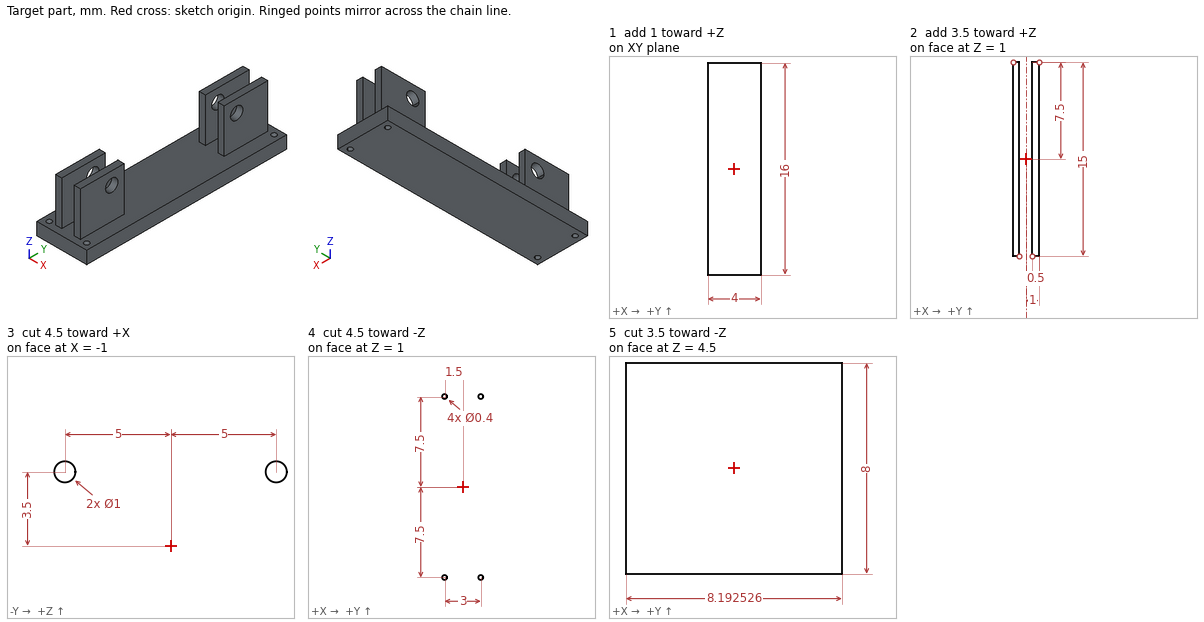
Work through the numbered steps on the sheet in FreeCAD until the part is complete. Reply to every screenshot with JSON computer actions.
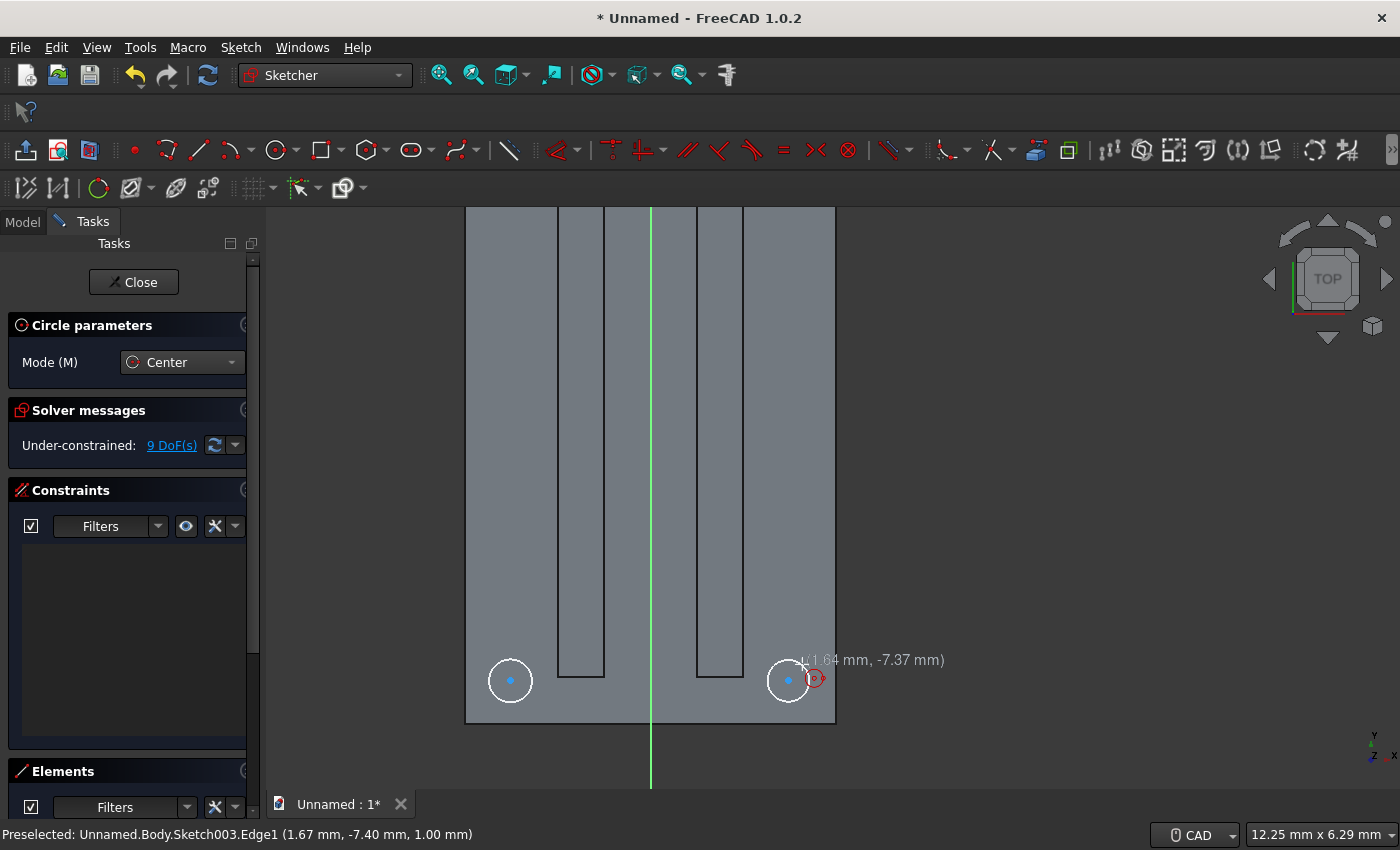
{"action": "scroll", "coordinate": [802, 666], "scroll_direction": "down", "scroll_amount": 7}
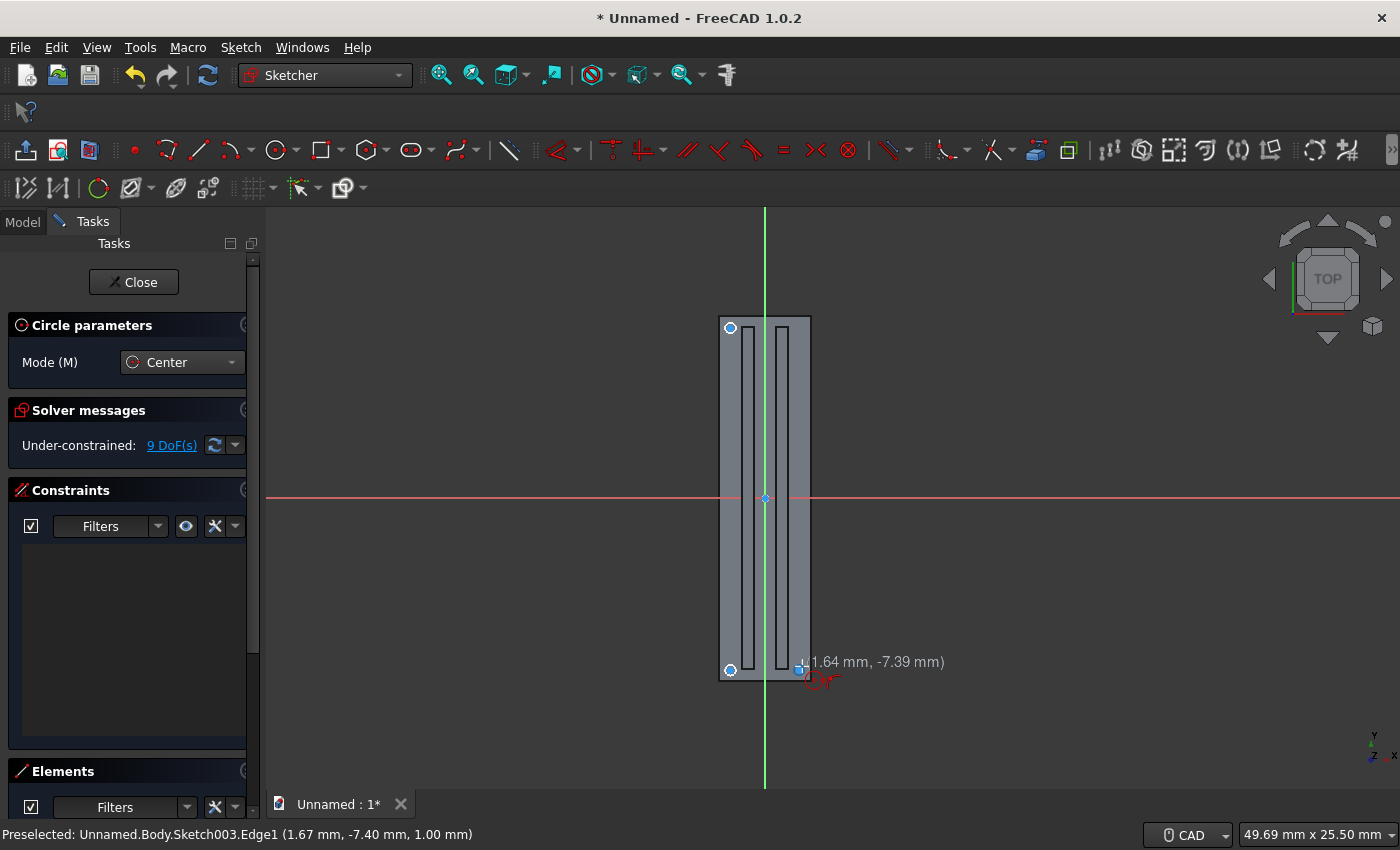
{"action": "scroll", "coordinate": [799, 327], "scroll_direction": "up", "scroll_amount": 9}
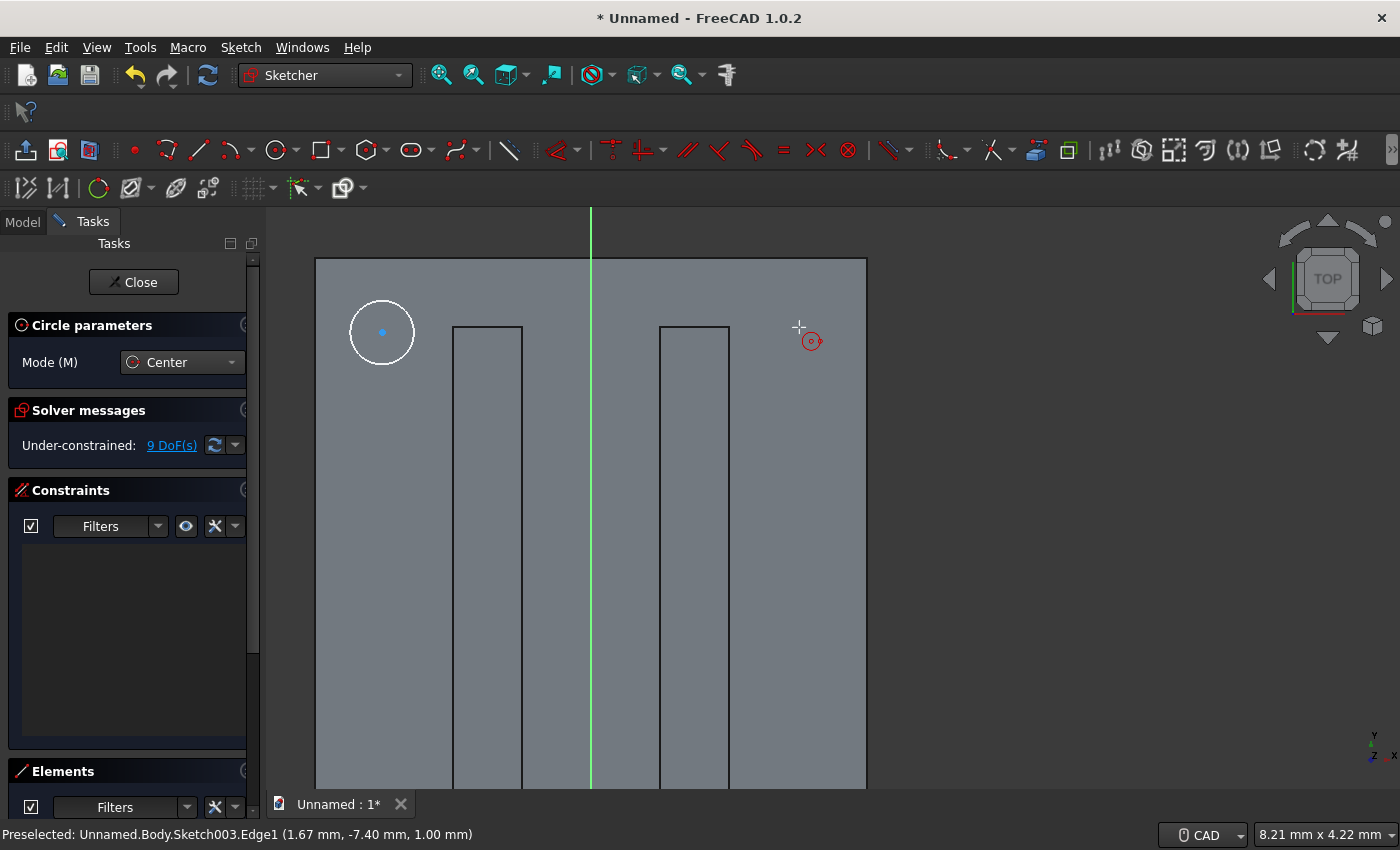
{"action": "scroll", "coordinate": [799, 327], "scroll_direction": "down", "scroll_amount": 9}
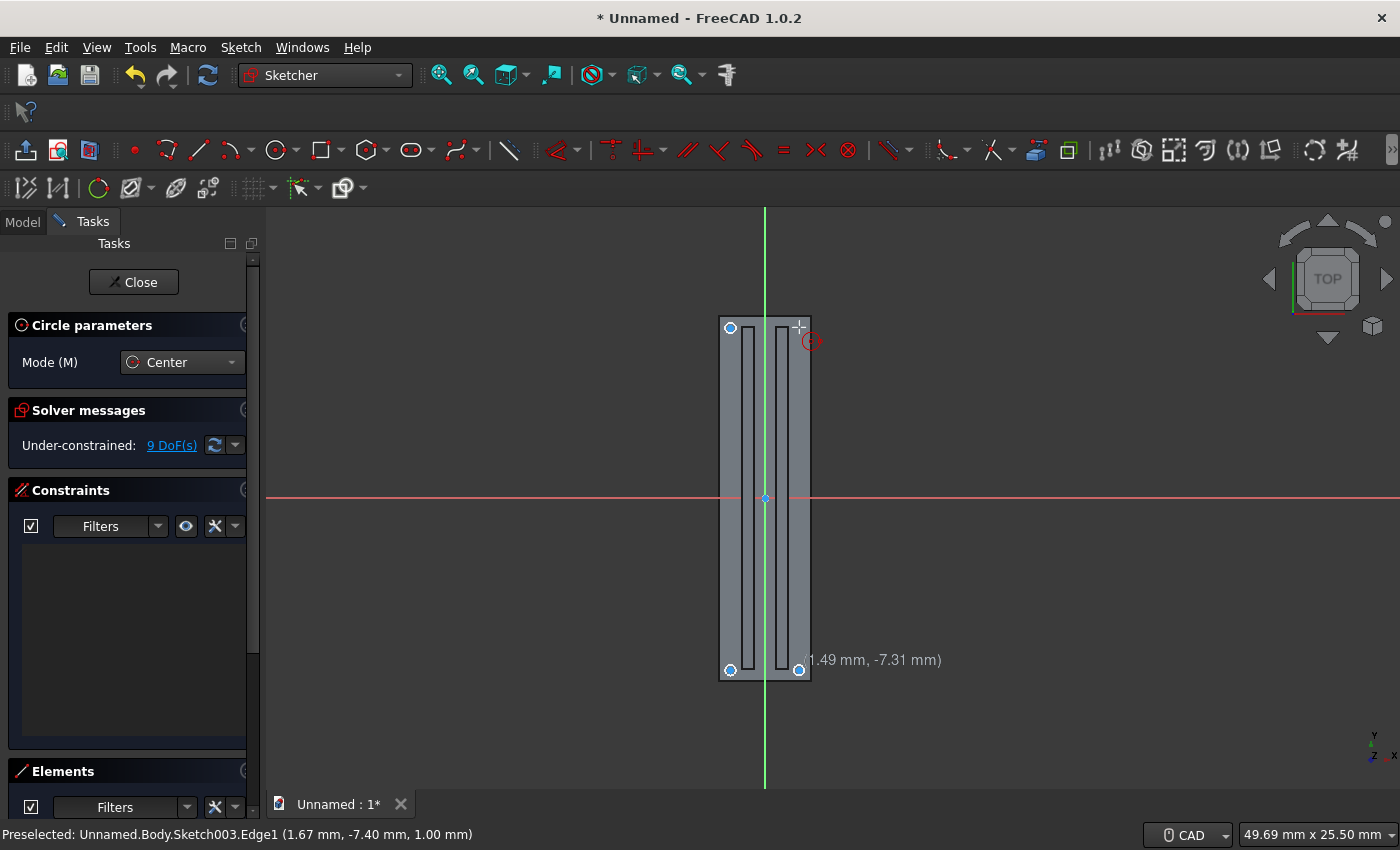
{"action": "left_click", "coordinate": [799, 327]}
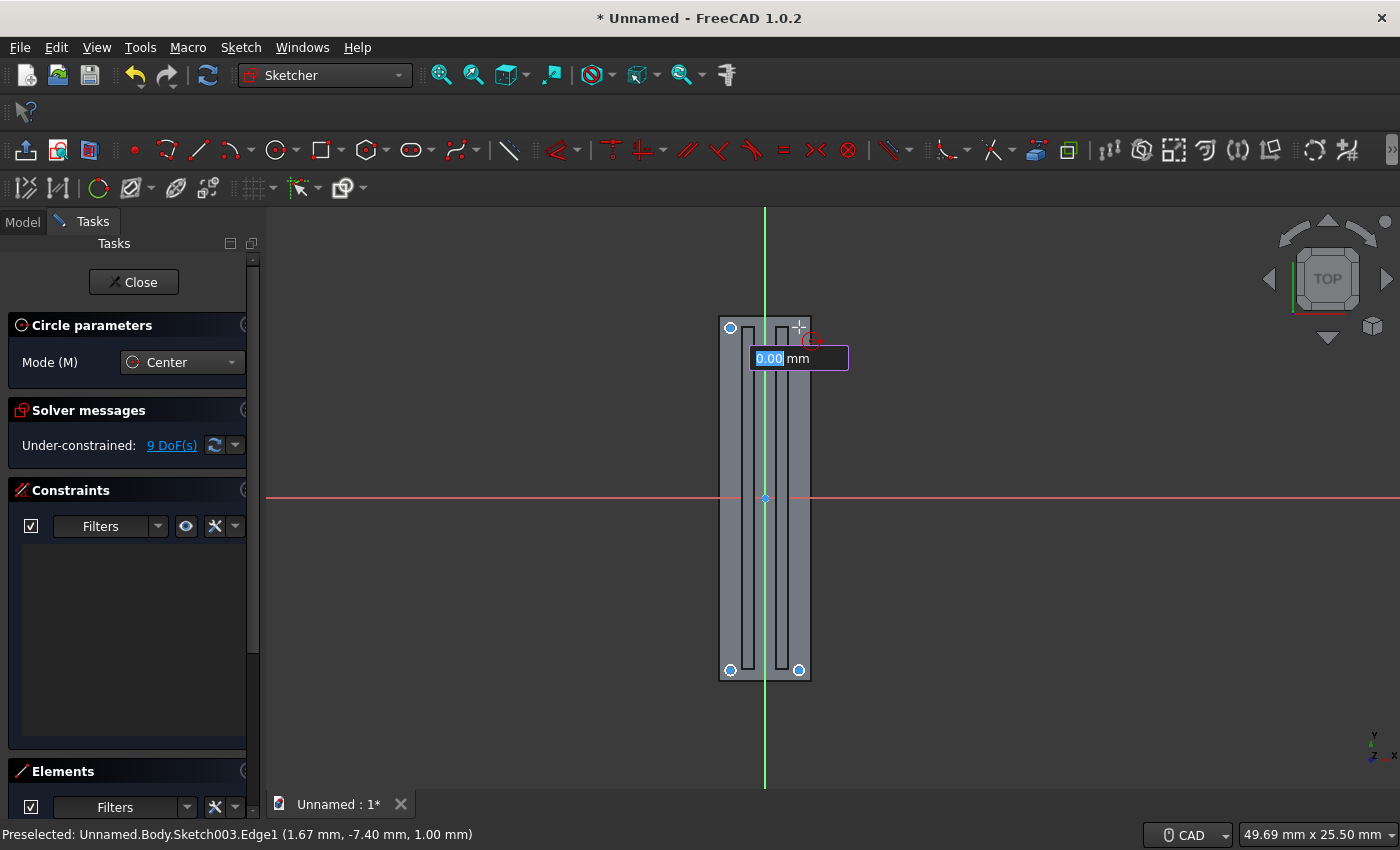
{"action": "scroll", "coordinate": [802, 324], "scroll_direction": "up", "scroll_amount": 7}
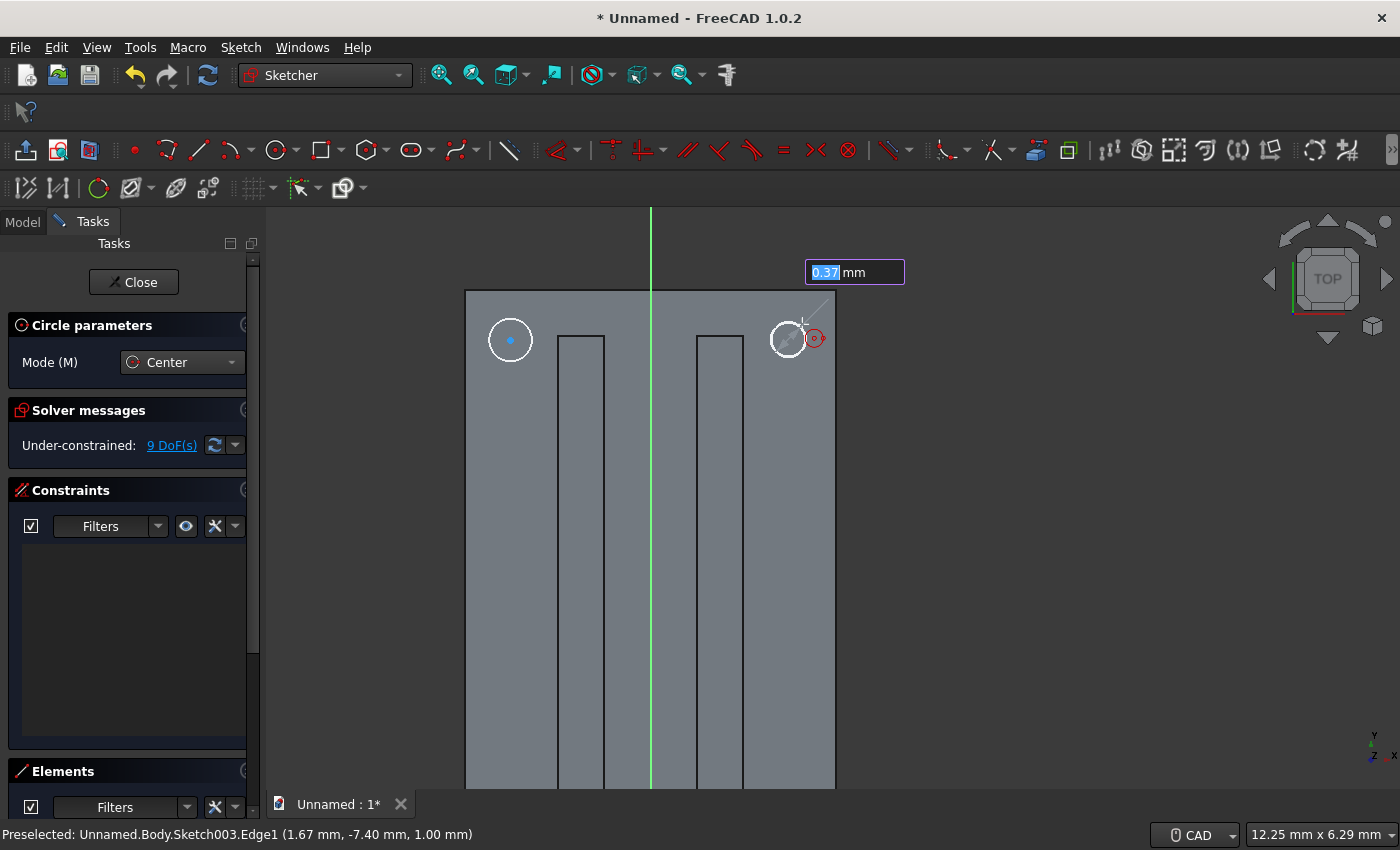
{"action": "left_click", "coordinate": [802, 323]}
{"action": "key", "text": "Escape"}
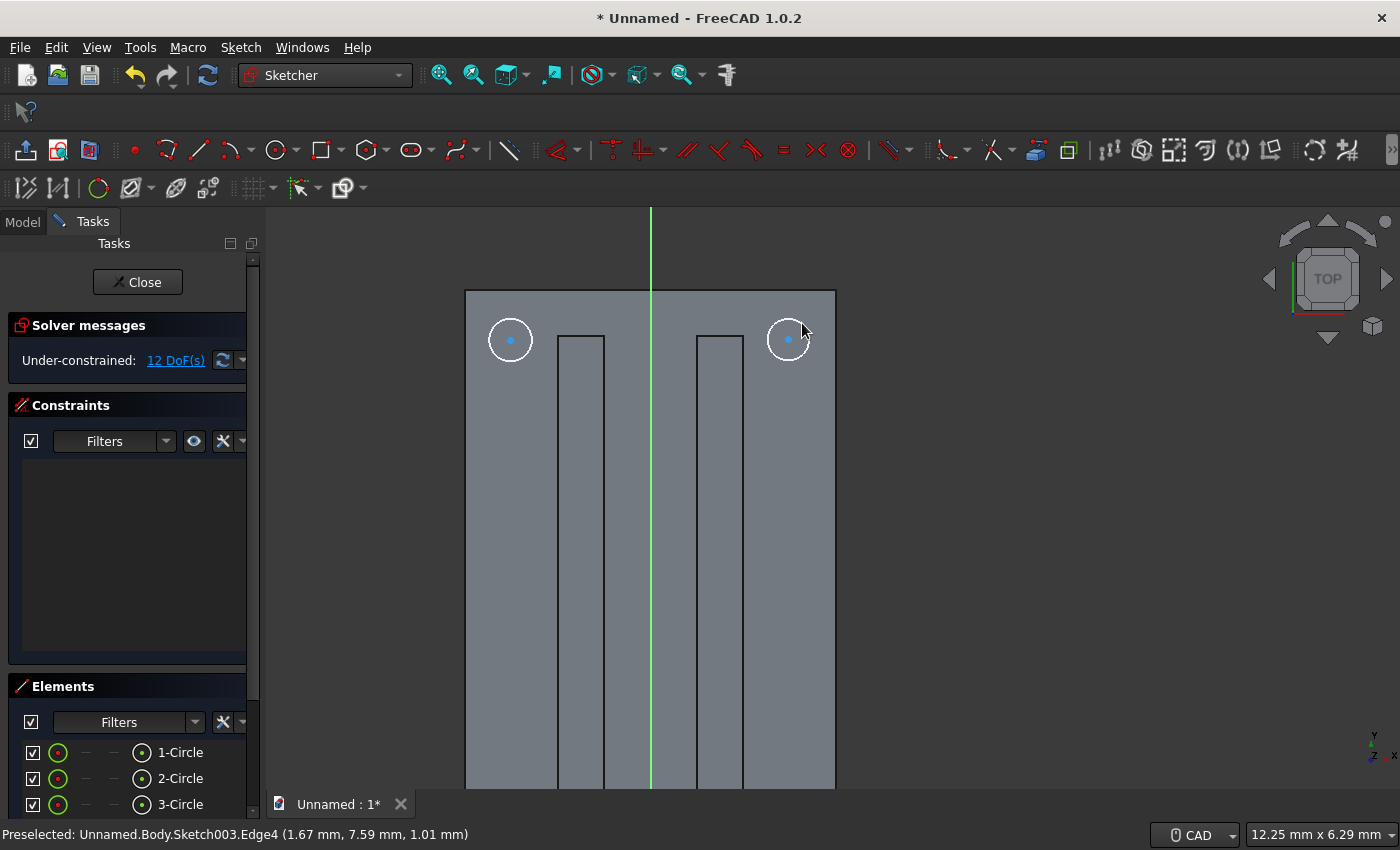
{"action": "left_click", "coordinate": [526, 325]}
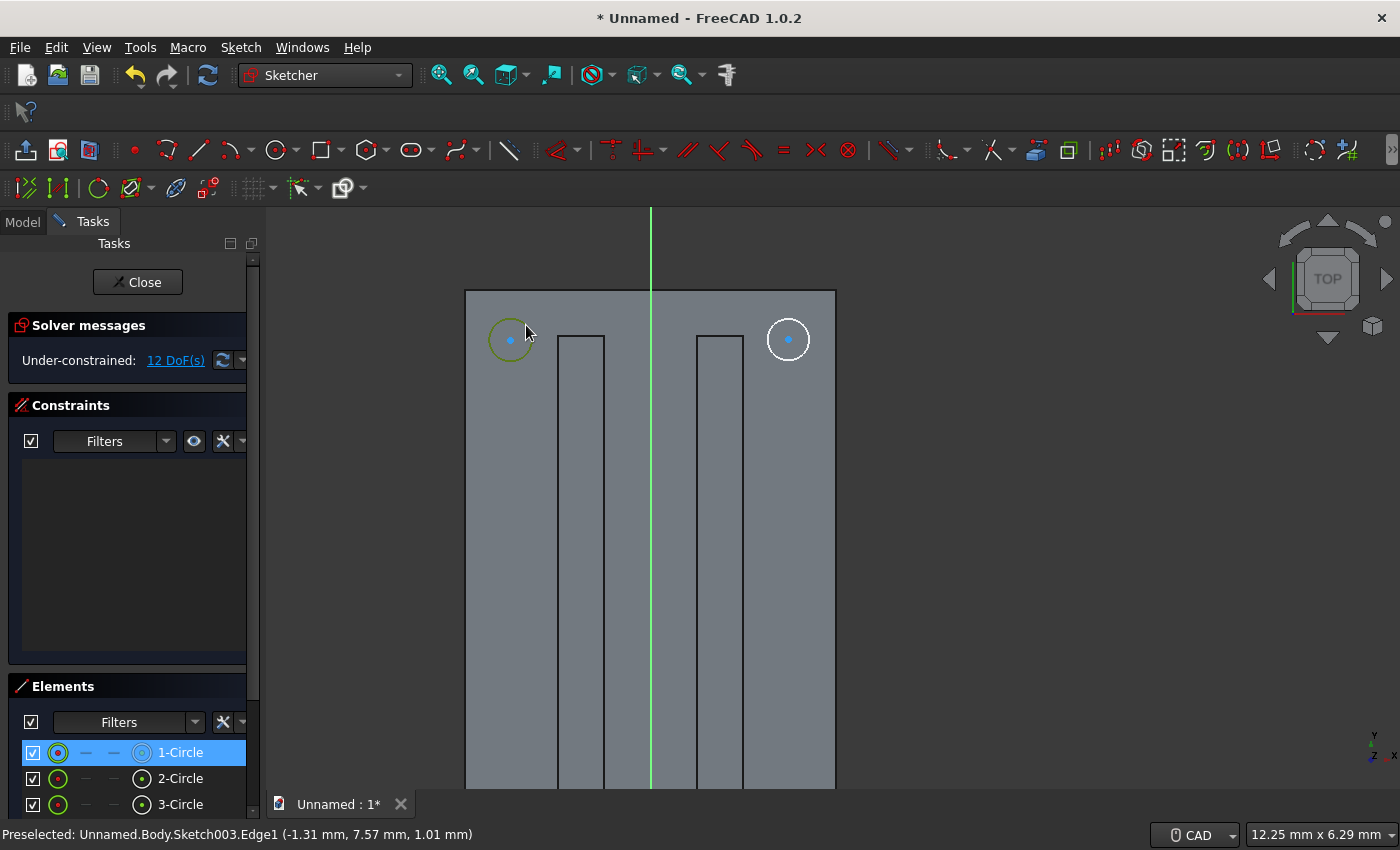
{"action": "scroll", "coordinate": [802, 324], "scroll_direction": "down", "scroll_amount": 7}